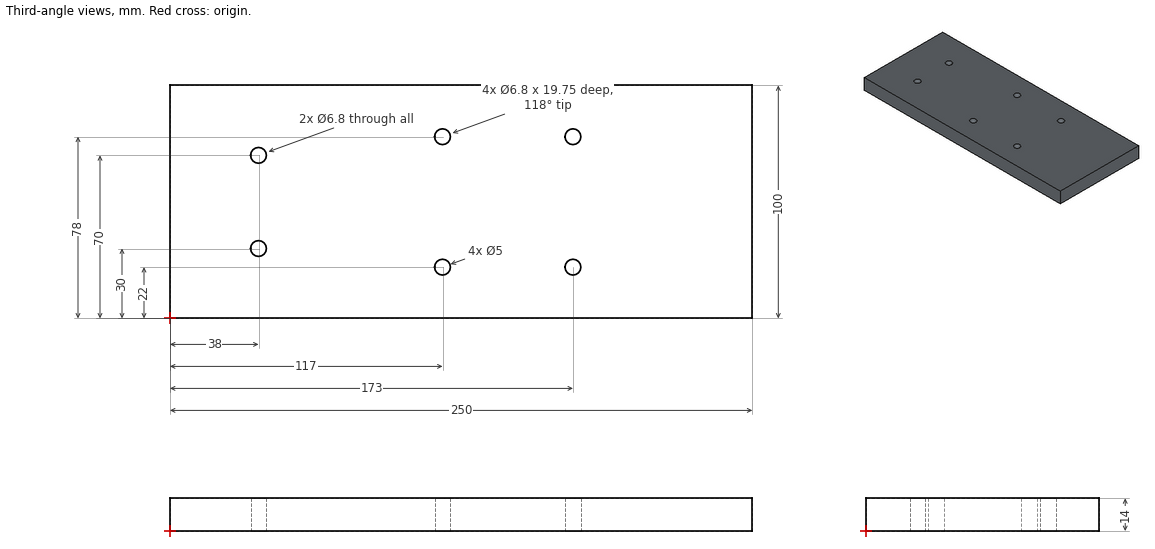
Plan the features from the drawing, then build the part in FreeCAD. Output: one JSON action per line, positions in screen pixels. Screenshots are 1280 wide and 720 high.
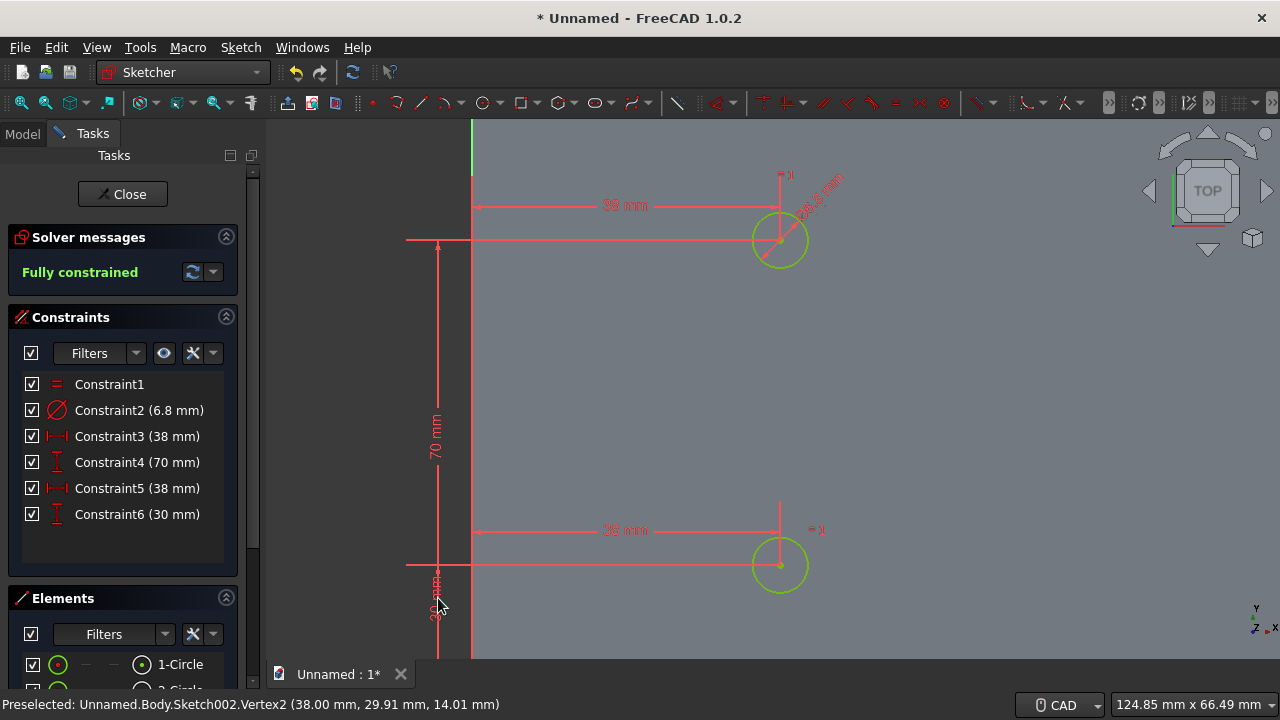
{"action": "left_click", "coordinate": [123, 194]}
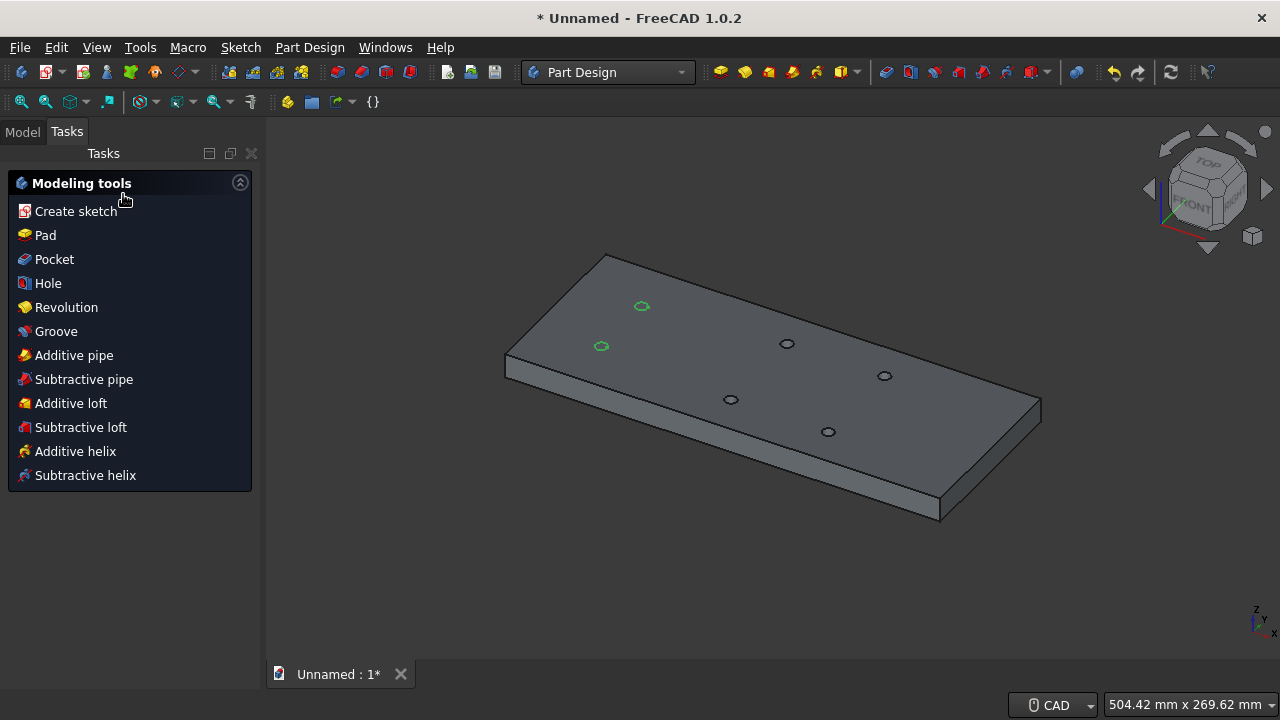
{"action": "left_click", "coordinate": [912, 72]}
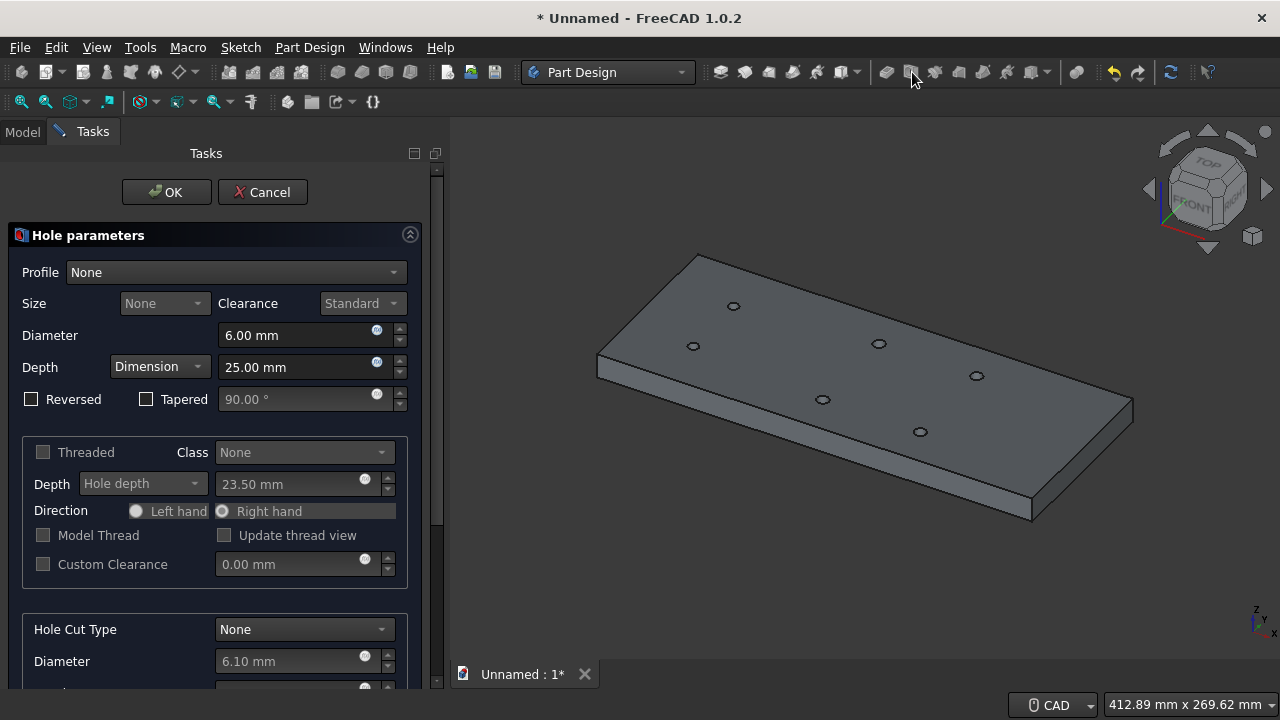
{"action": "triple_click", "coordinate": [305, 335]}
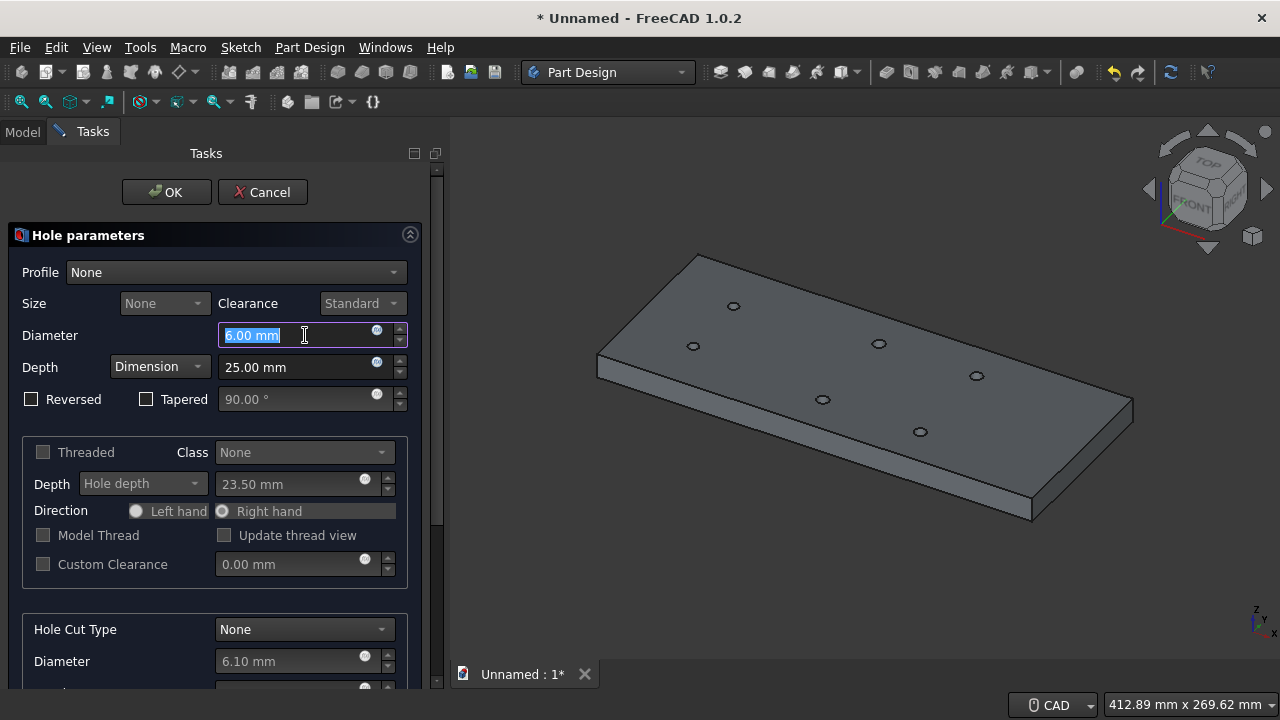
{"action": "type", "text": "6.8"}
{"action": "key", "text": "Tab"}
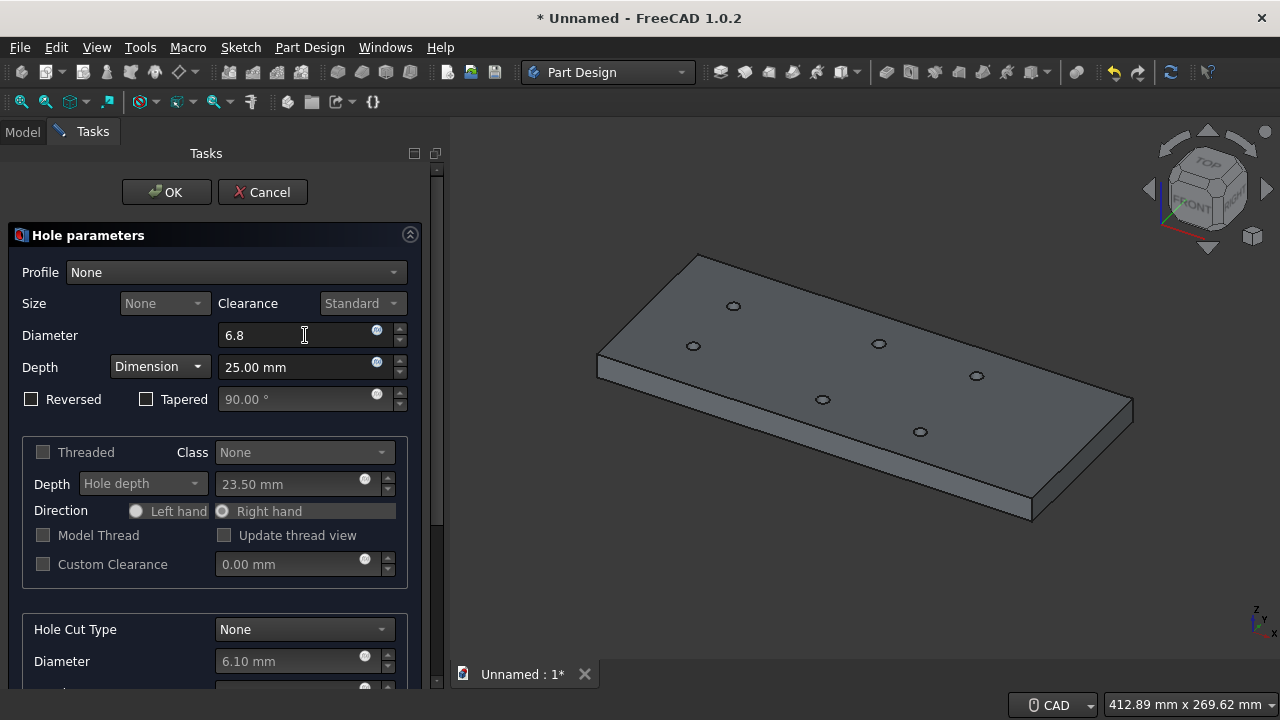
{"action": "left_click", "coordinate": [161, 366]}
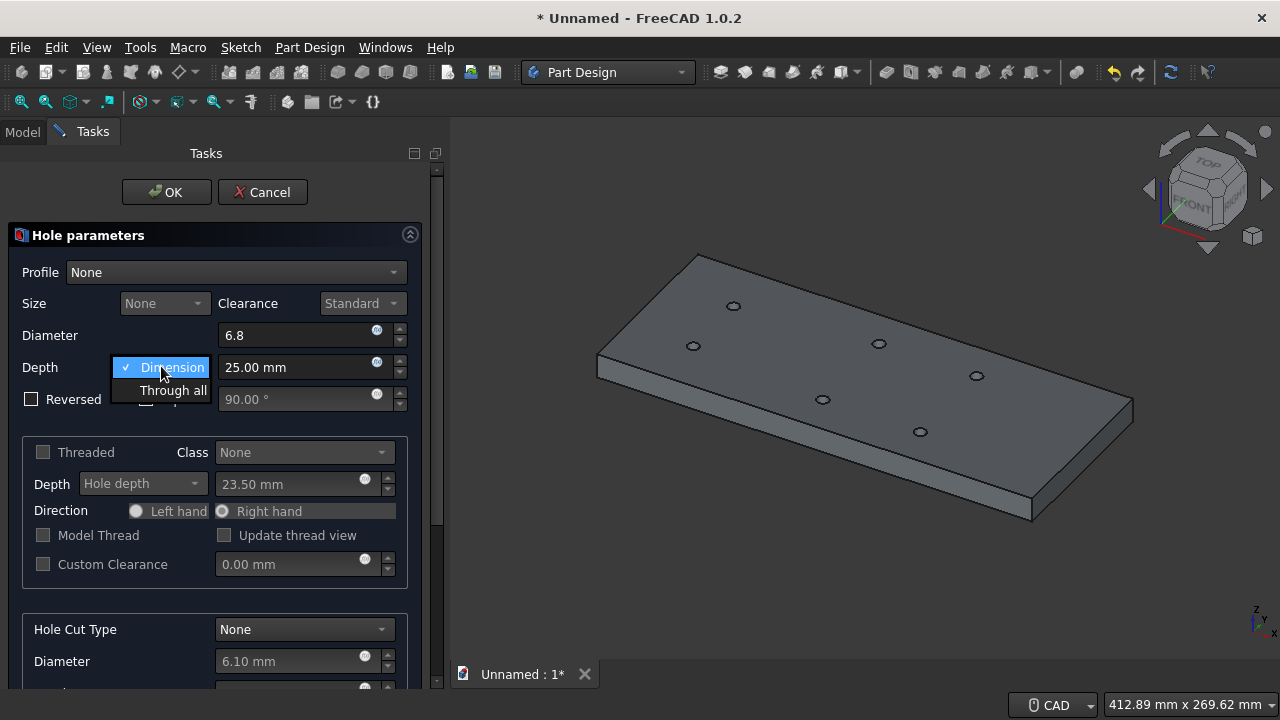
{"action": "left_click", "coordinate": [160, 390]}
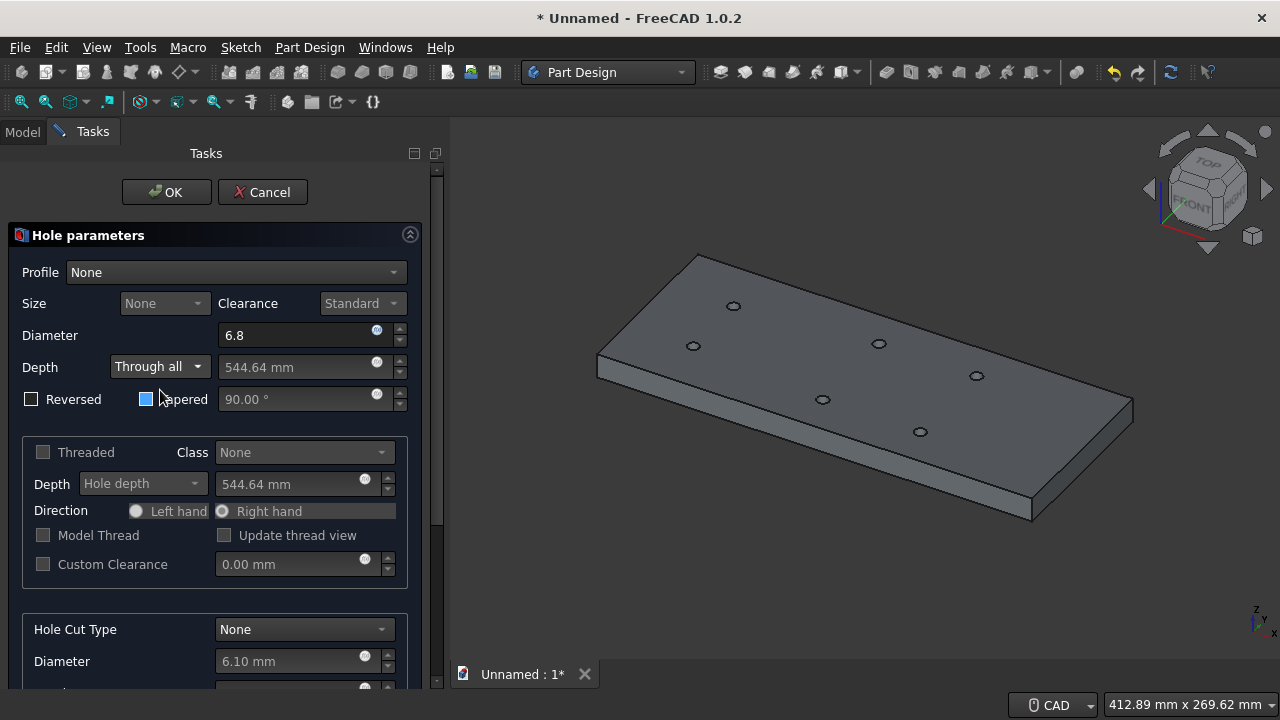
{"action": "left_click", "coordinate": [167, 192]}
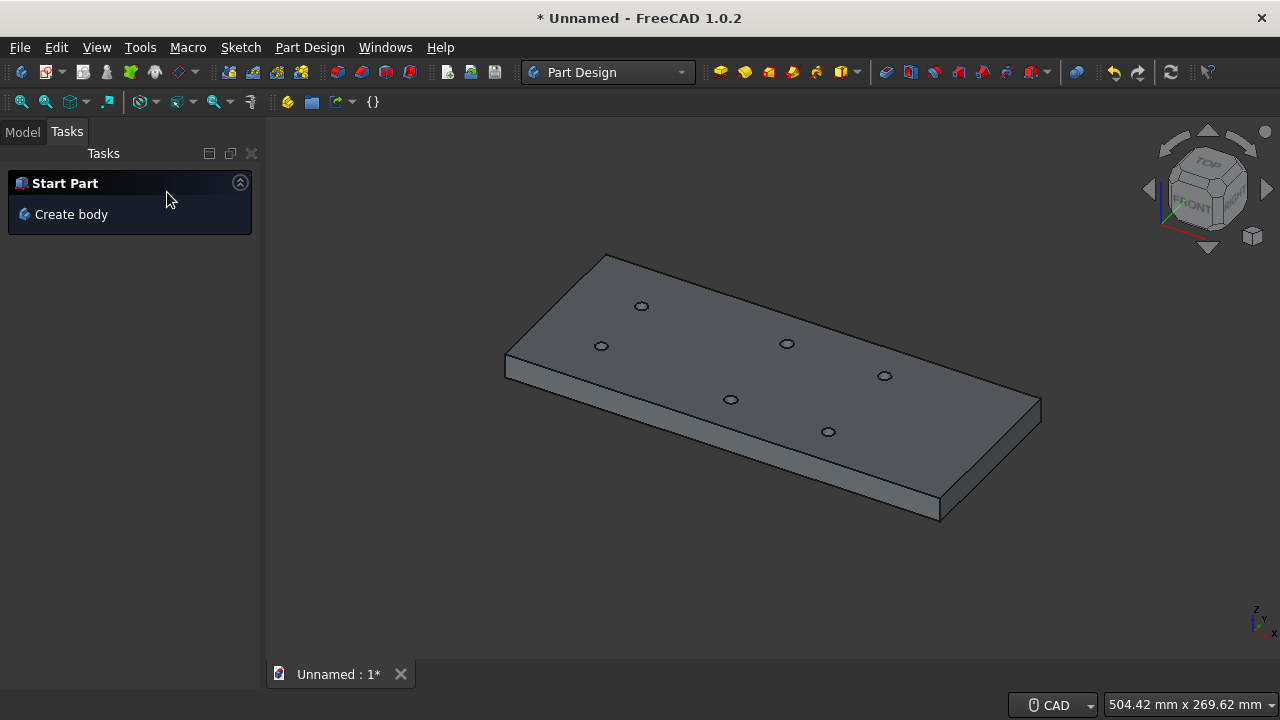
{"action": "key", "text": "0"}